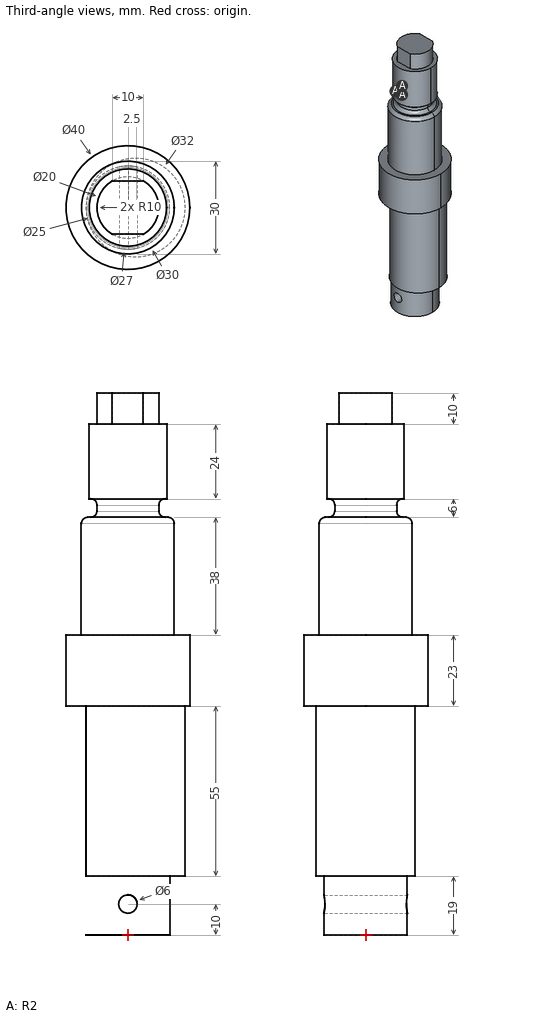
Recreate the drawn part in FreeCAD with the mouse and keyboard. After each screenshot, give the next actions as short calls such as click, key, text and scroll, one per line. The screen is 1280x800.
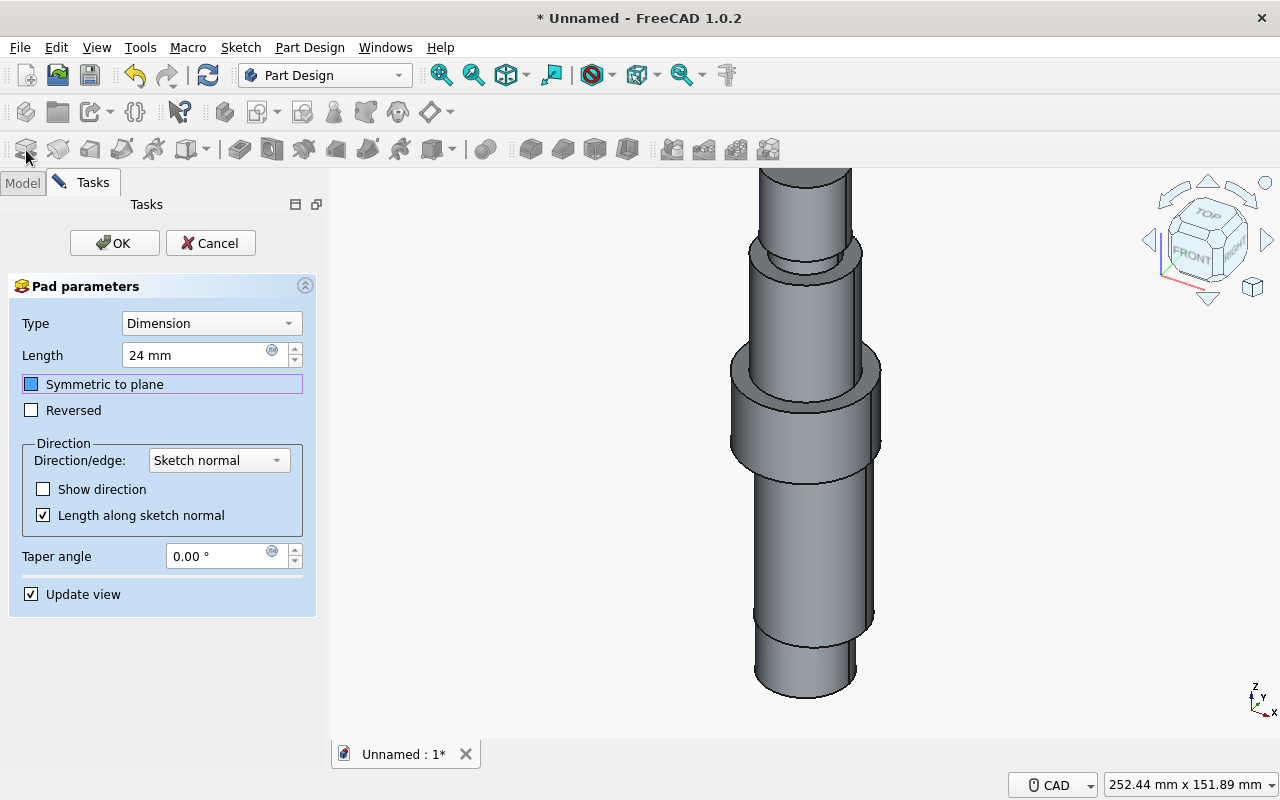
click(115, 243)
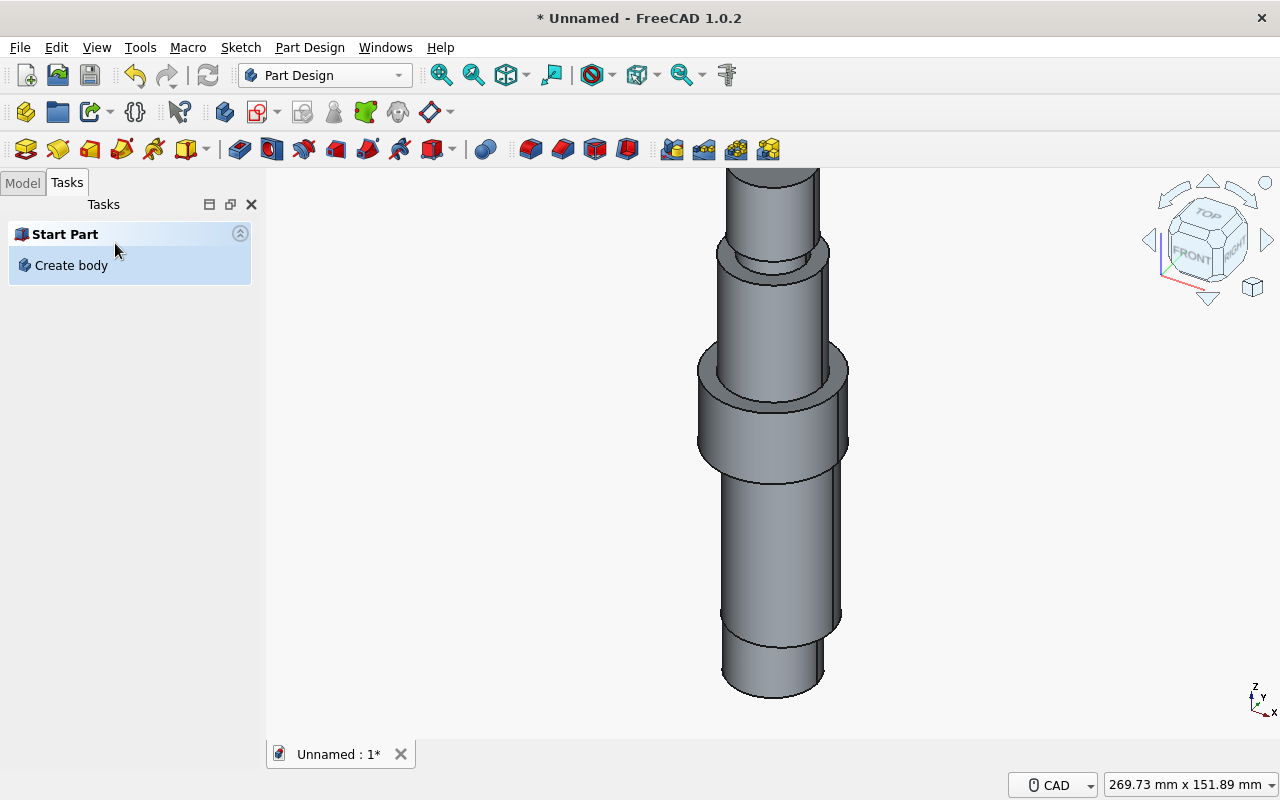
key(v)
key(f)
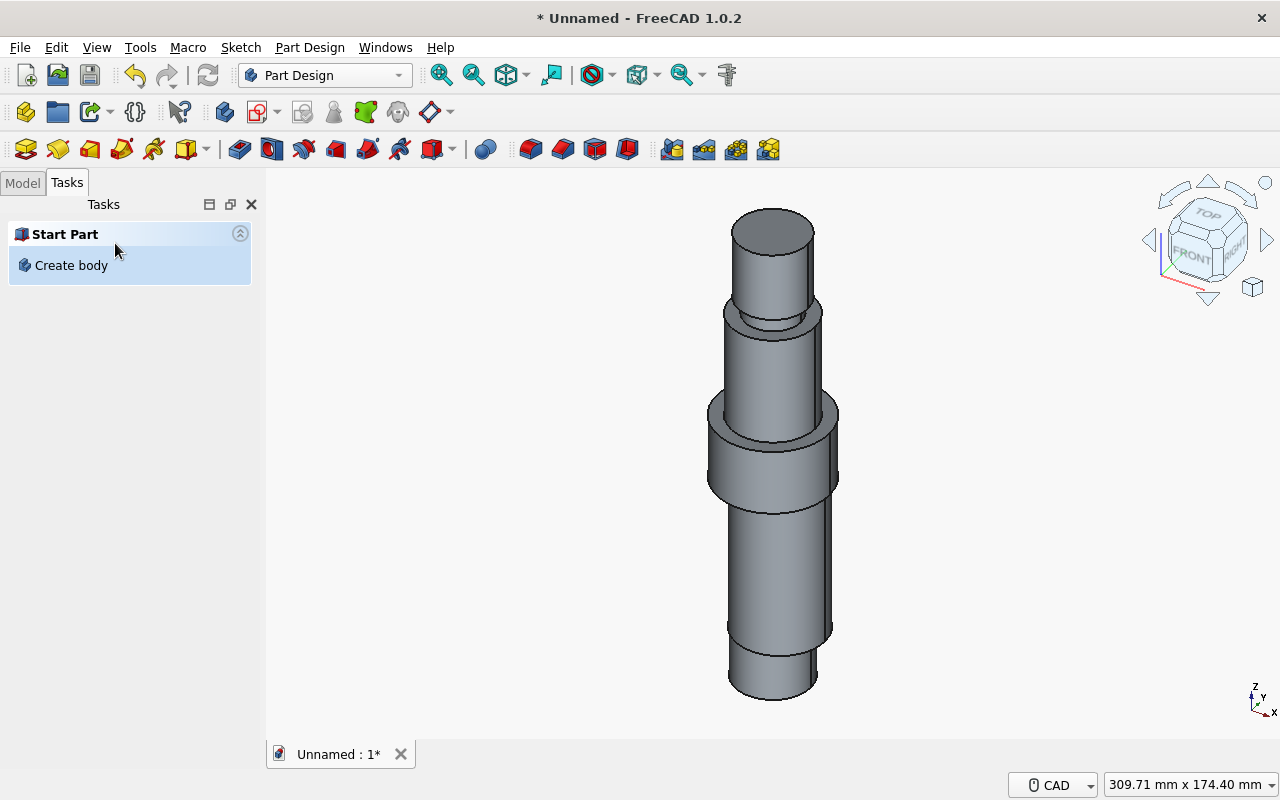
click(773, 231)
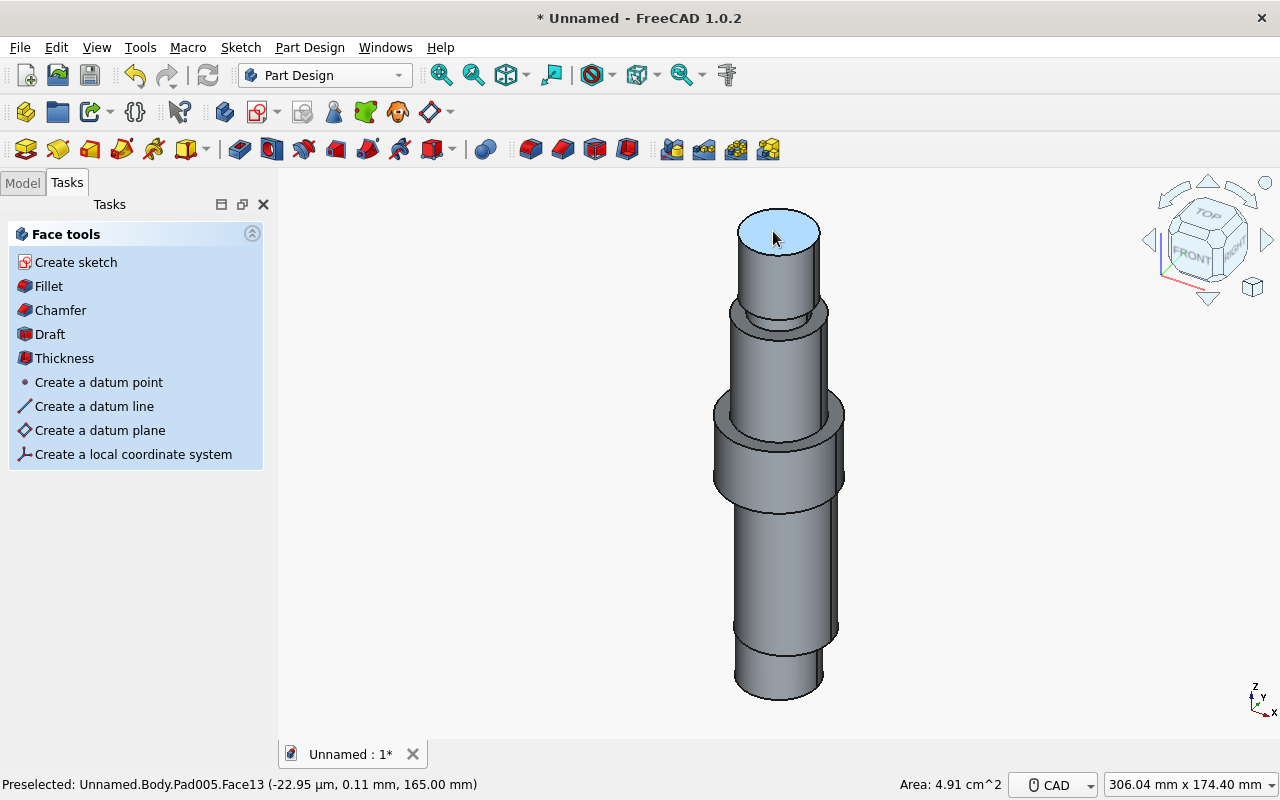
click(258, 112)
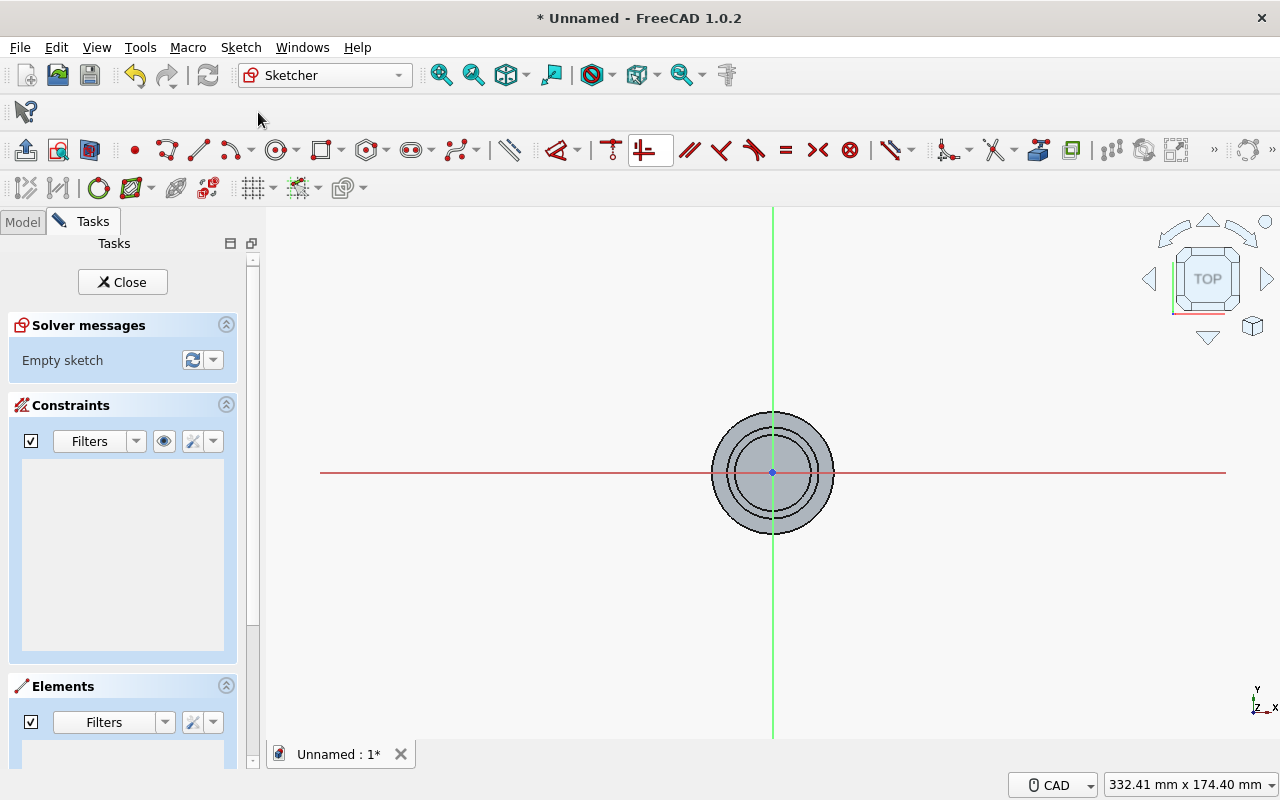
scroll(786, 473, up, 9)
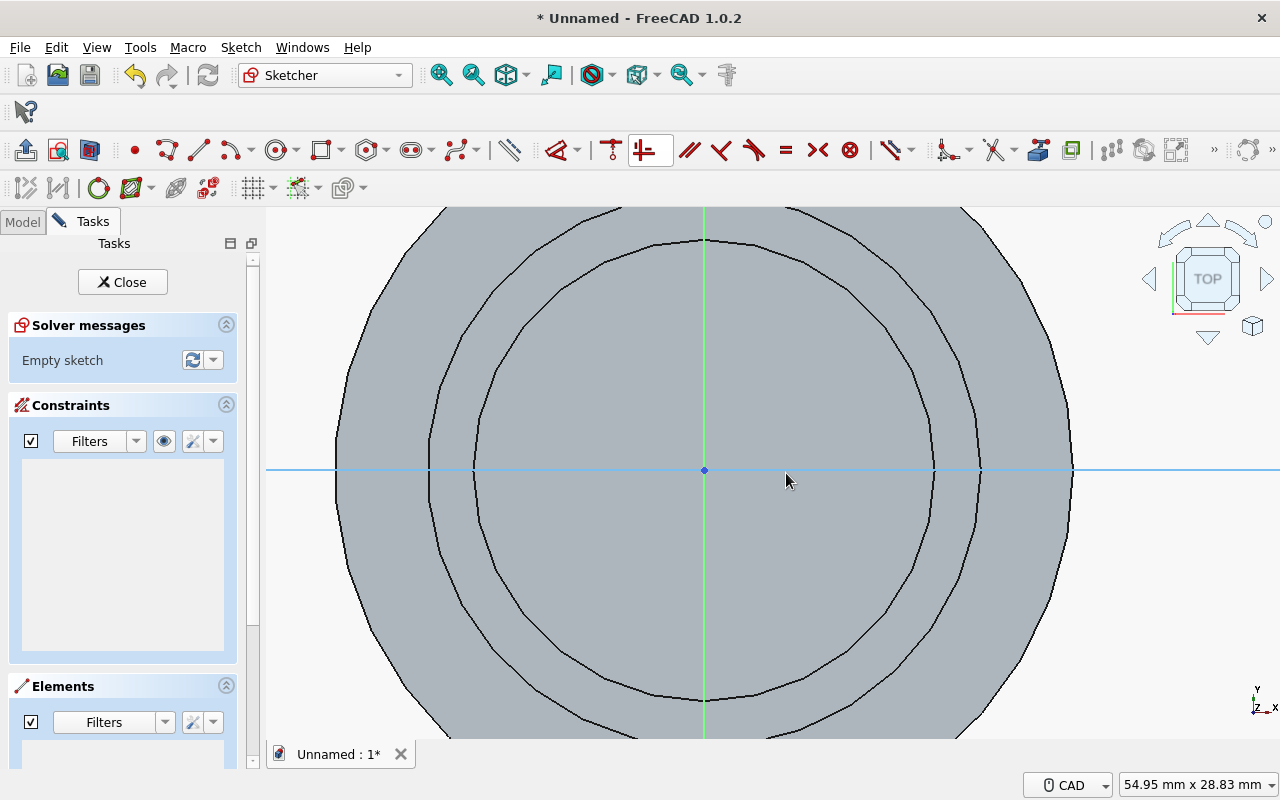
key(g)
key(l)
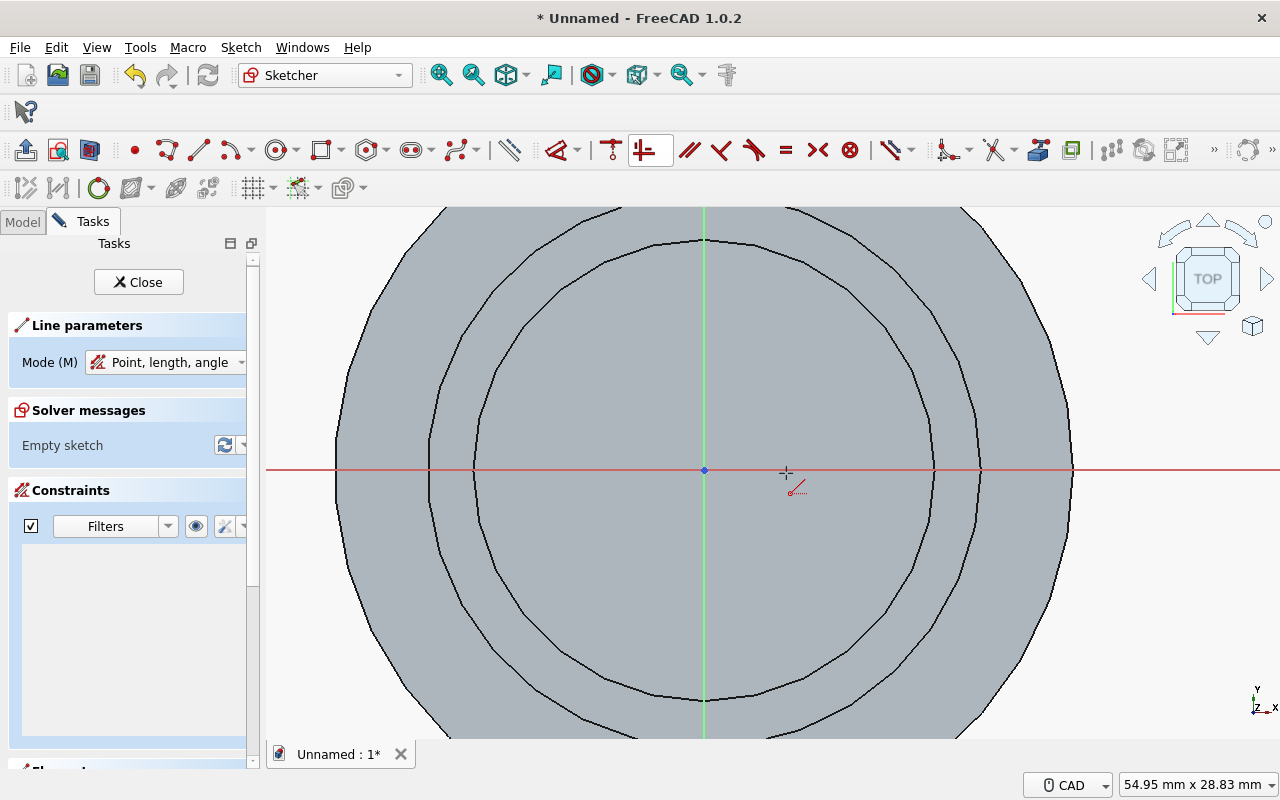
click(796, 311)
click(612, 311)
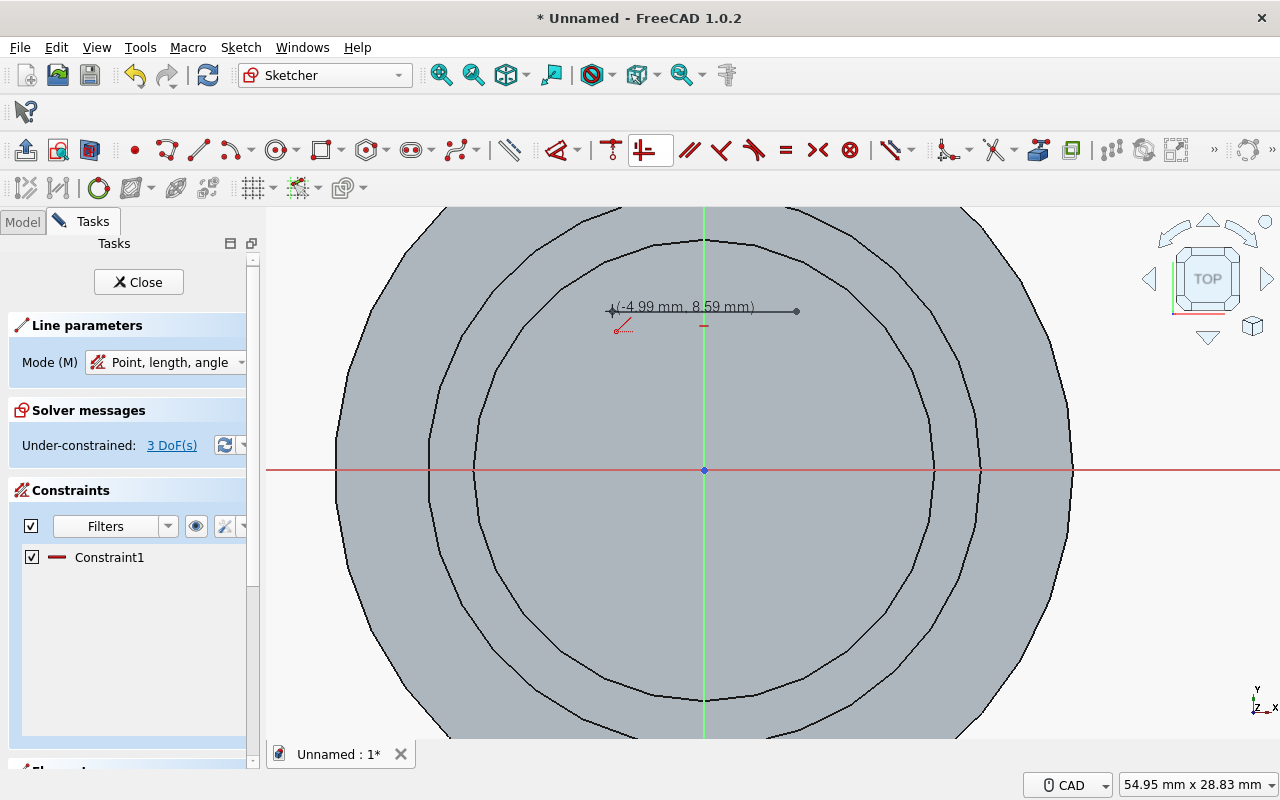
click(612, 630)
click(796, 630)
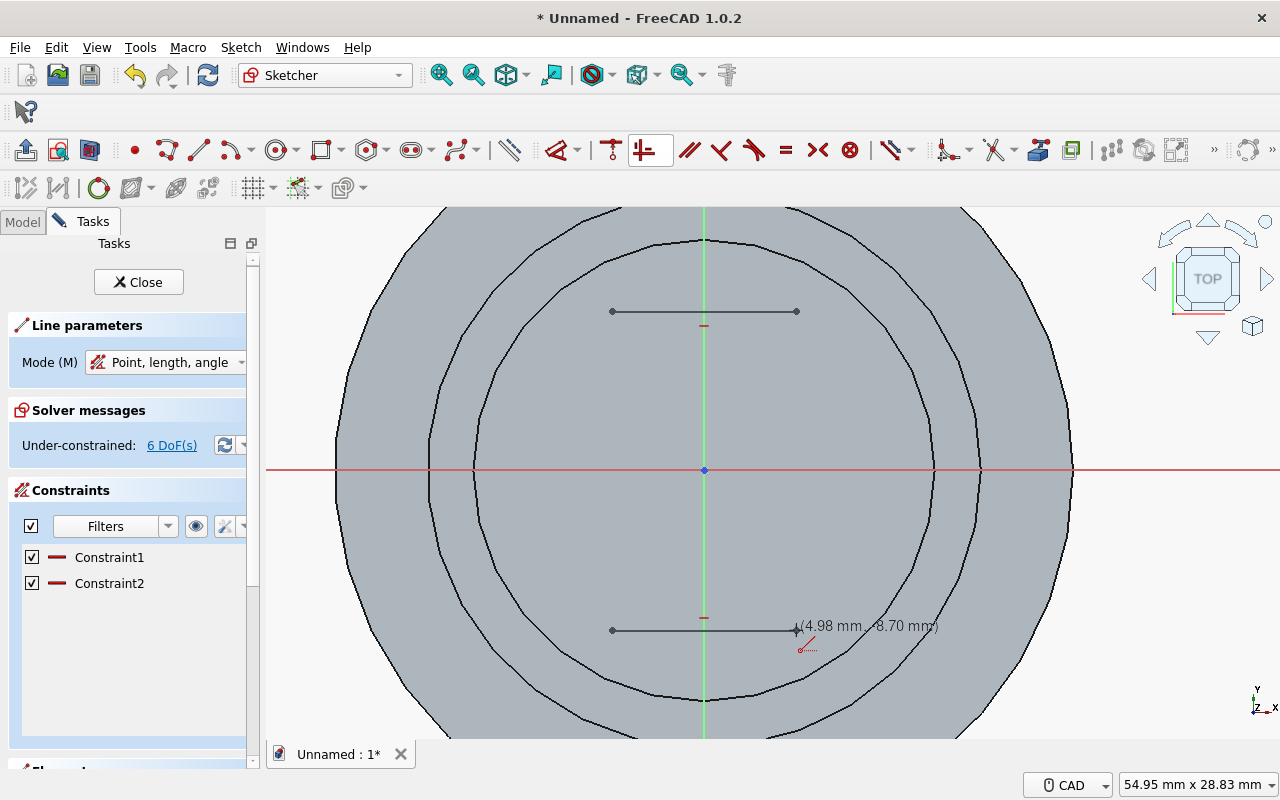
key(g)
key(3)
key(a)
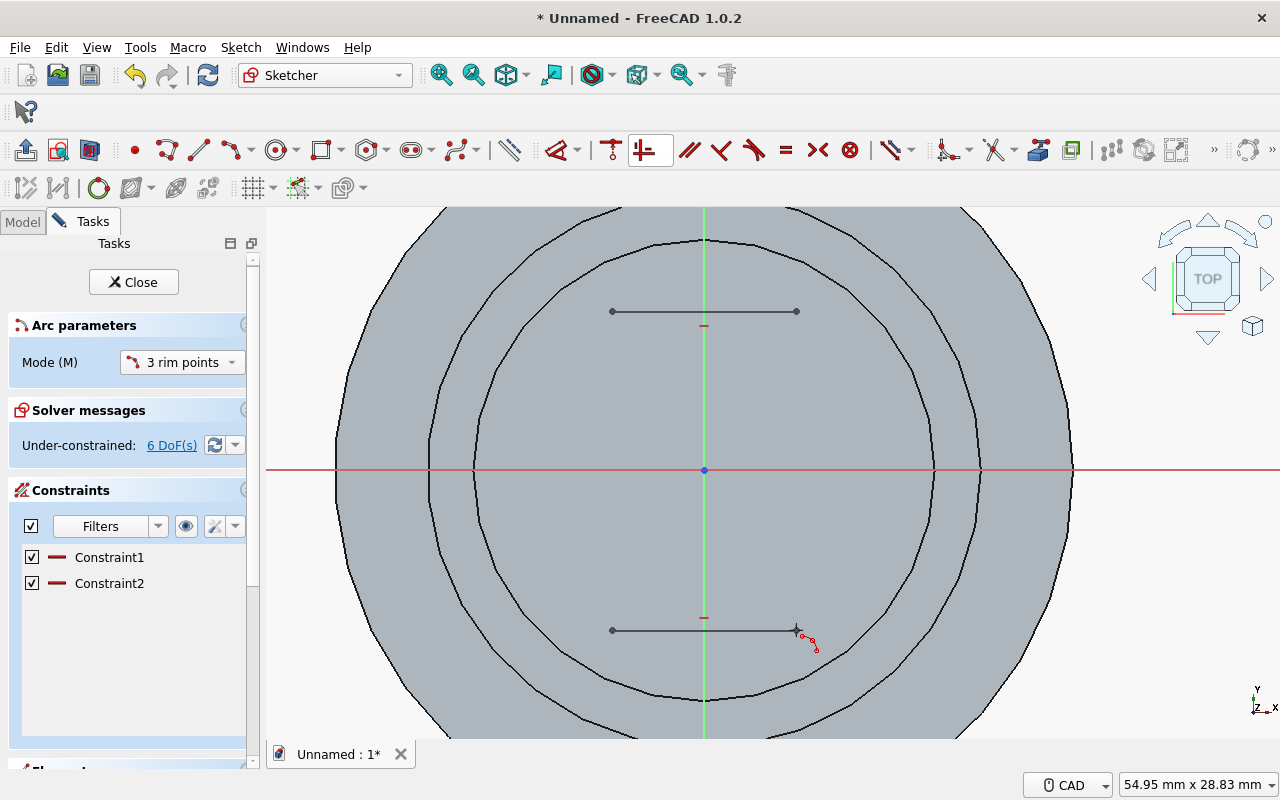
click(612, 312)
click(612, 631)
click(524, 432)